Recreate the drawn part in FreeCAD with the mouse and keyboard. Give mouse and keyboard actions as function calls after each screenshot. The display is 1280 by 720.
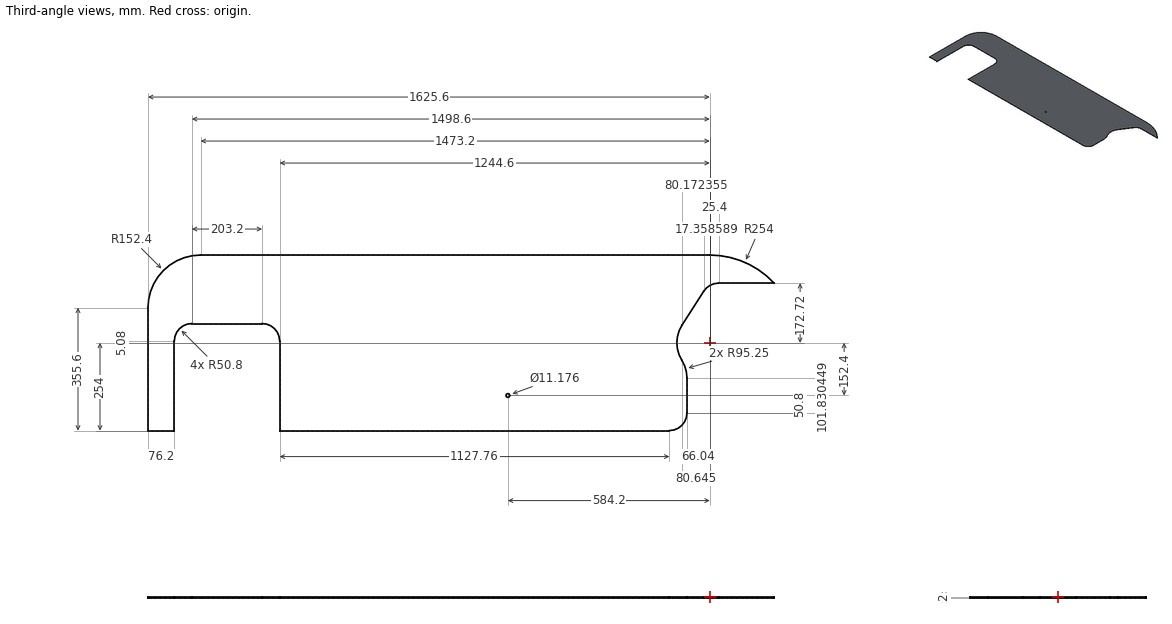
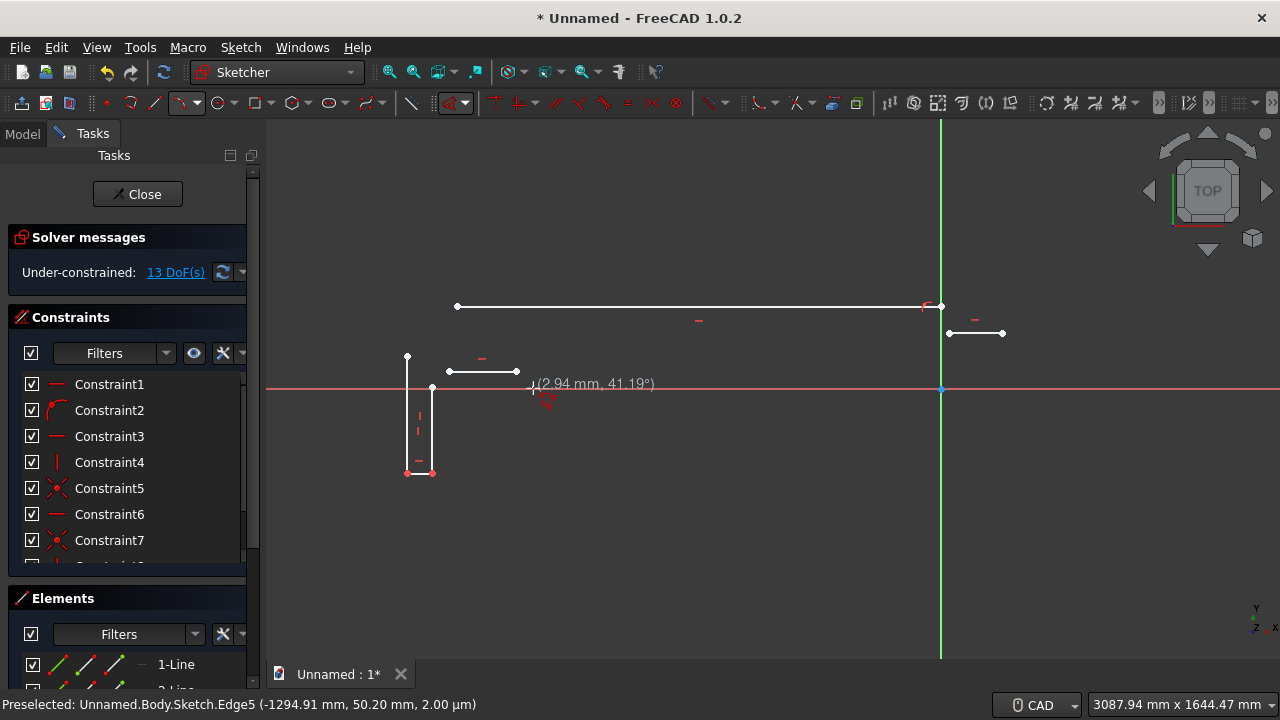
click(533, 473)
click(903, 473)
right_click(903, 473)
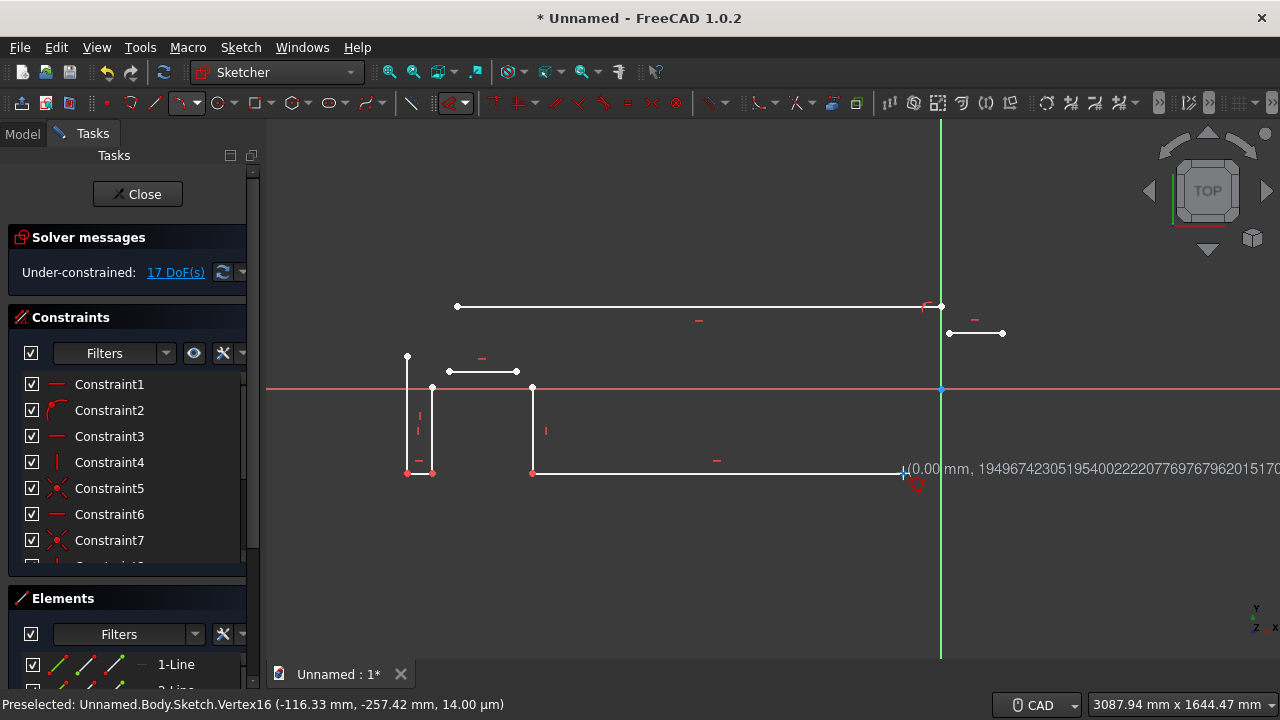
click(156, 104)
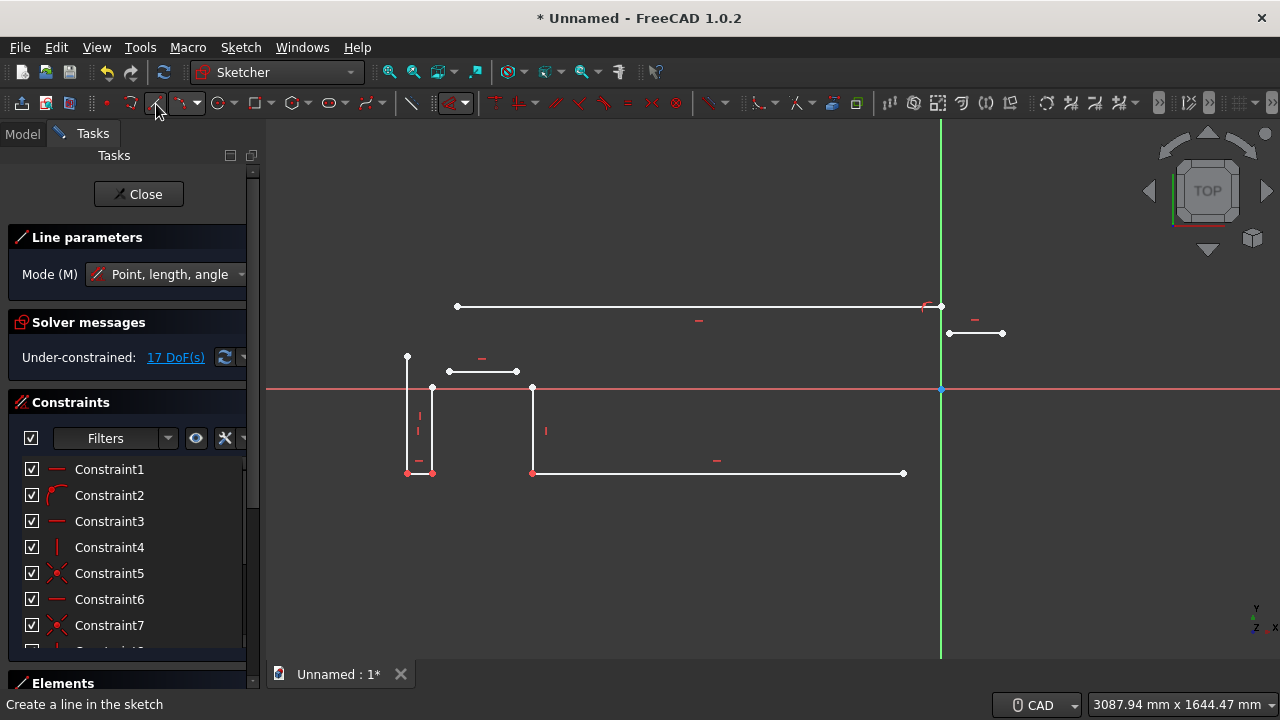
click(920, 456)
click(920, 423)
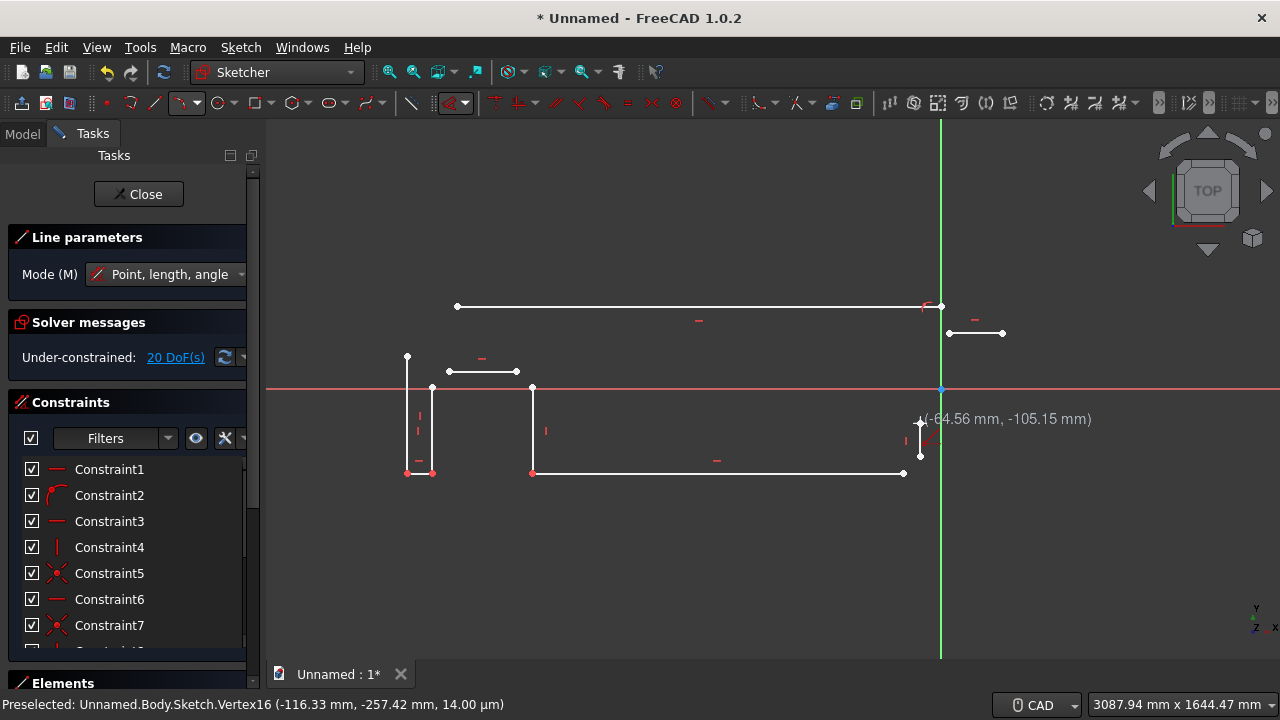
click(915, 373)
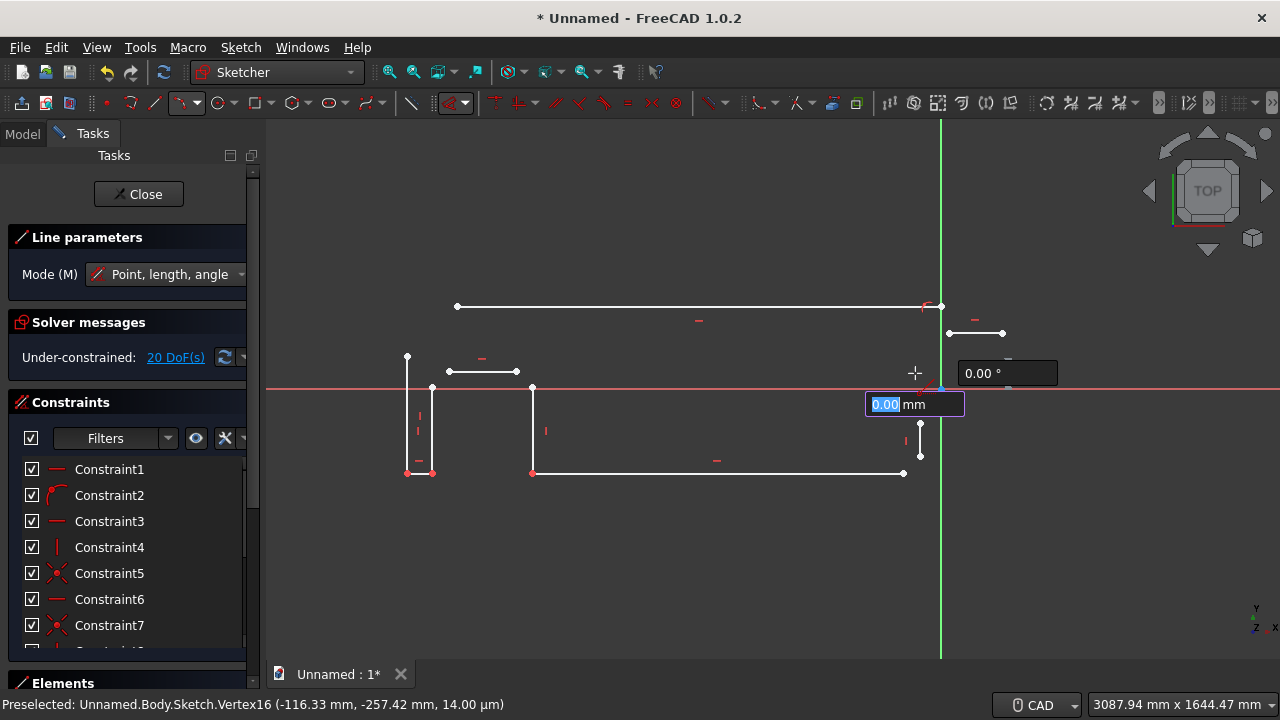
scroll(935, 340, up, 6)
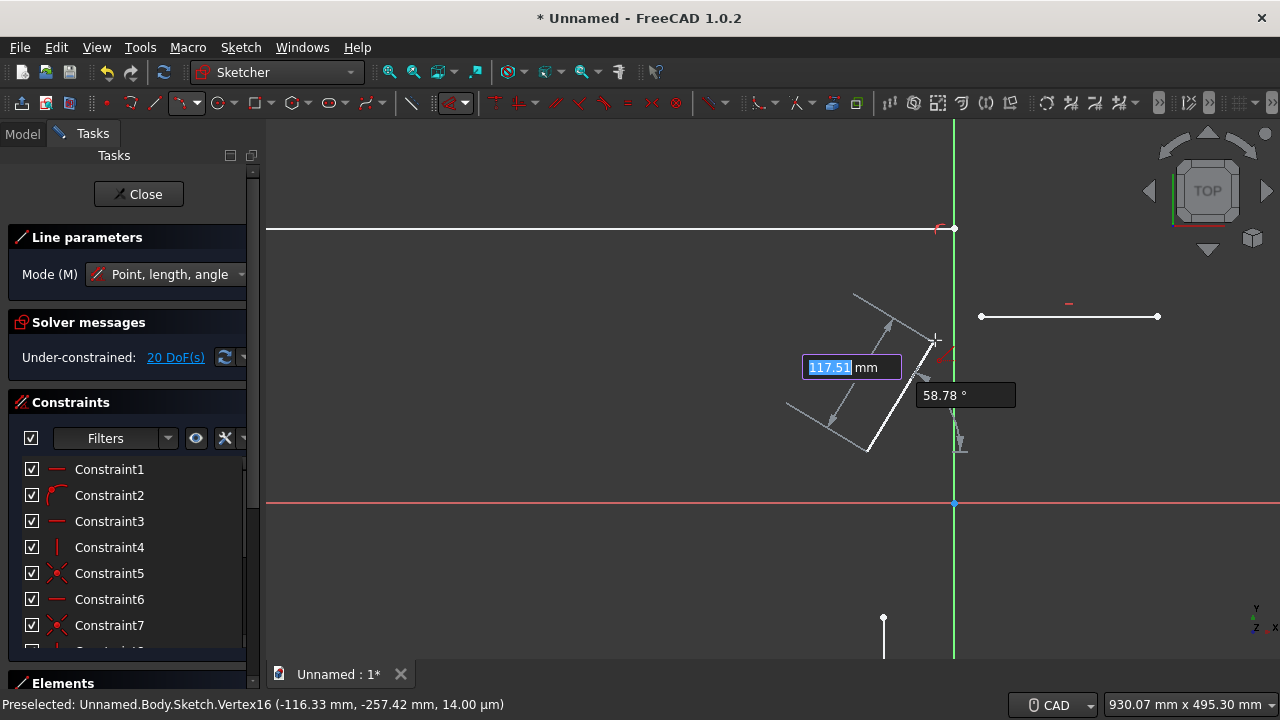
click(935, 340)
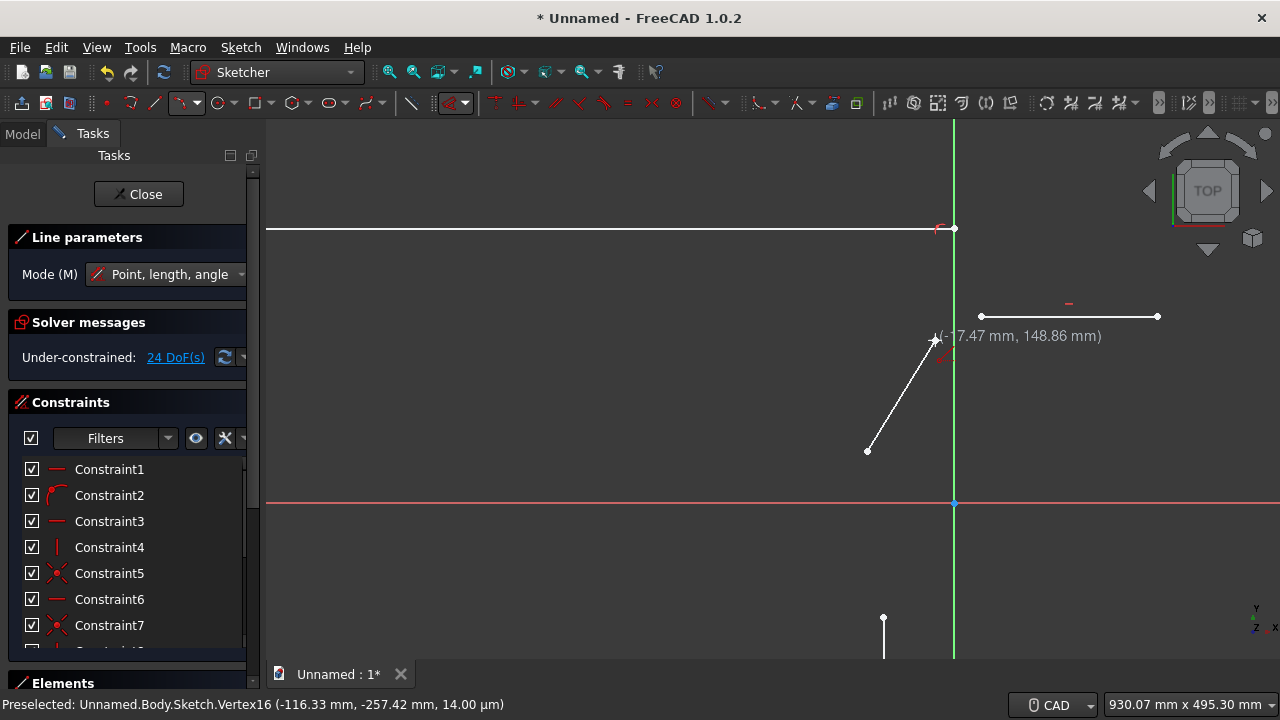
click(180, 104)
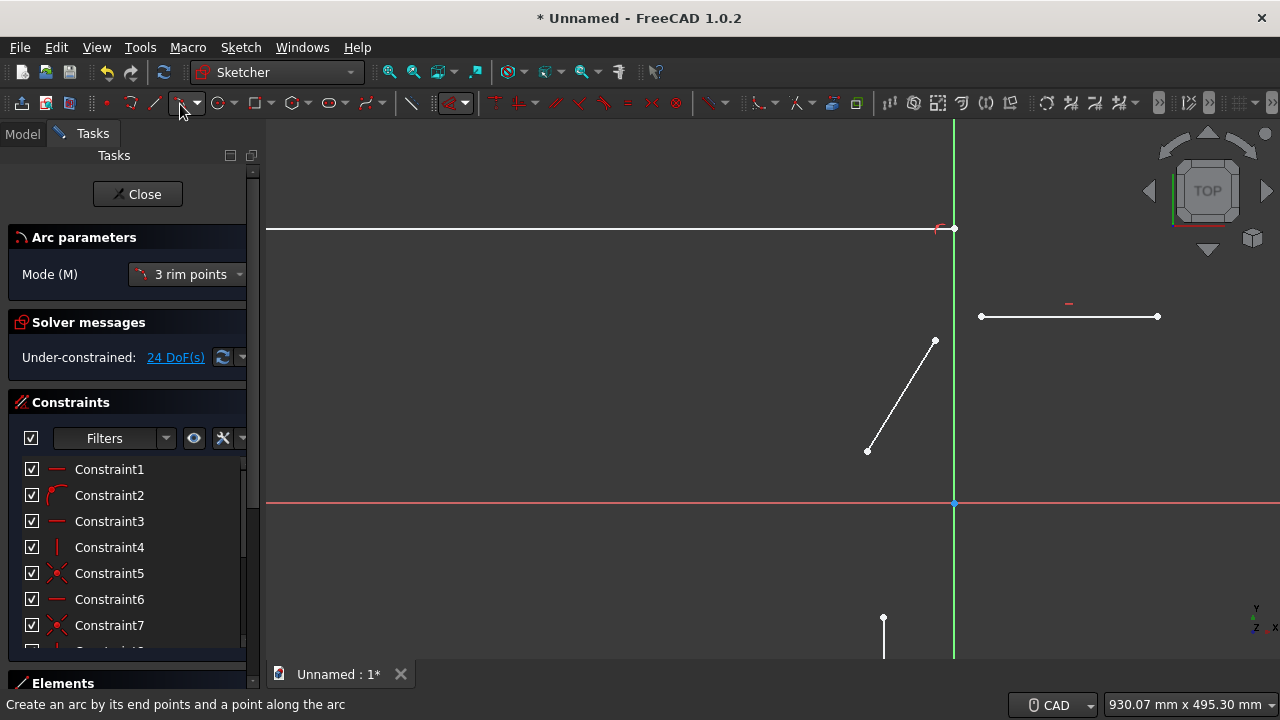
scroll(935, 340, down, 6)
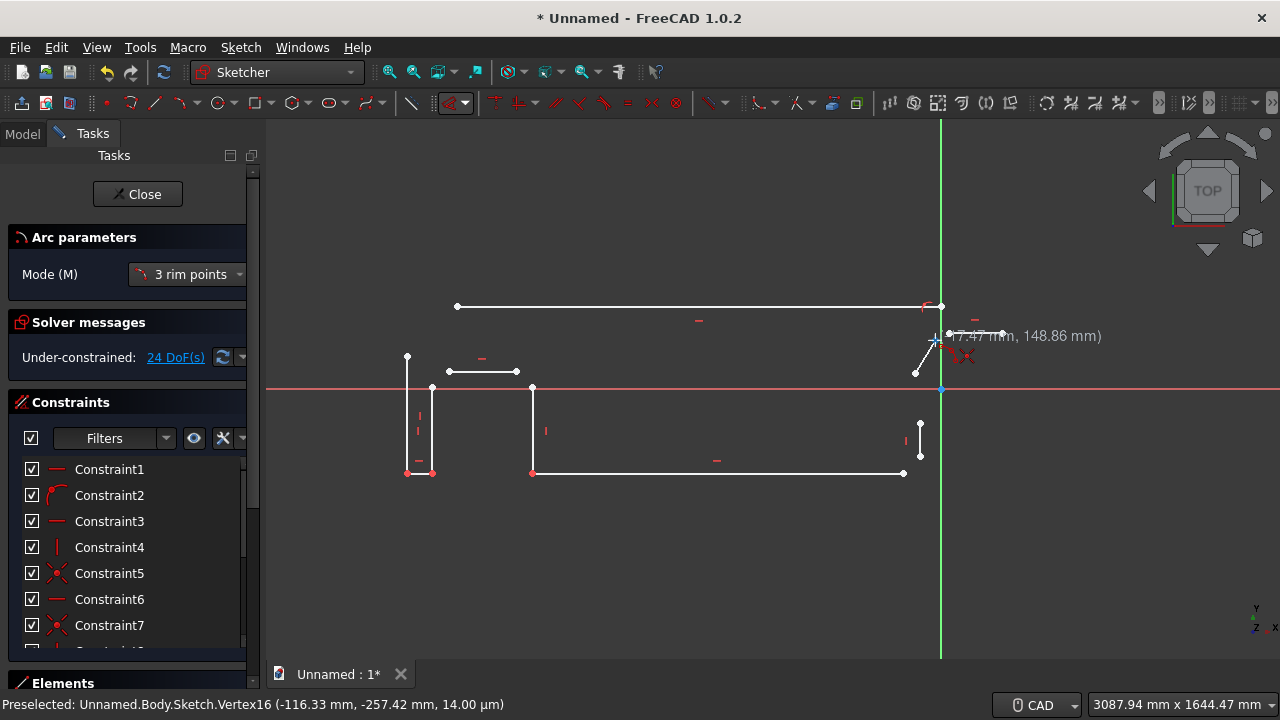
click(1002, 333)
click(941, 307)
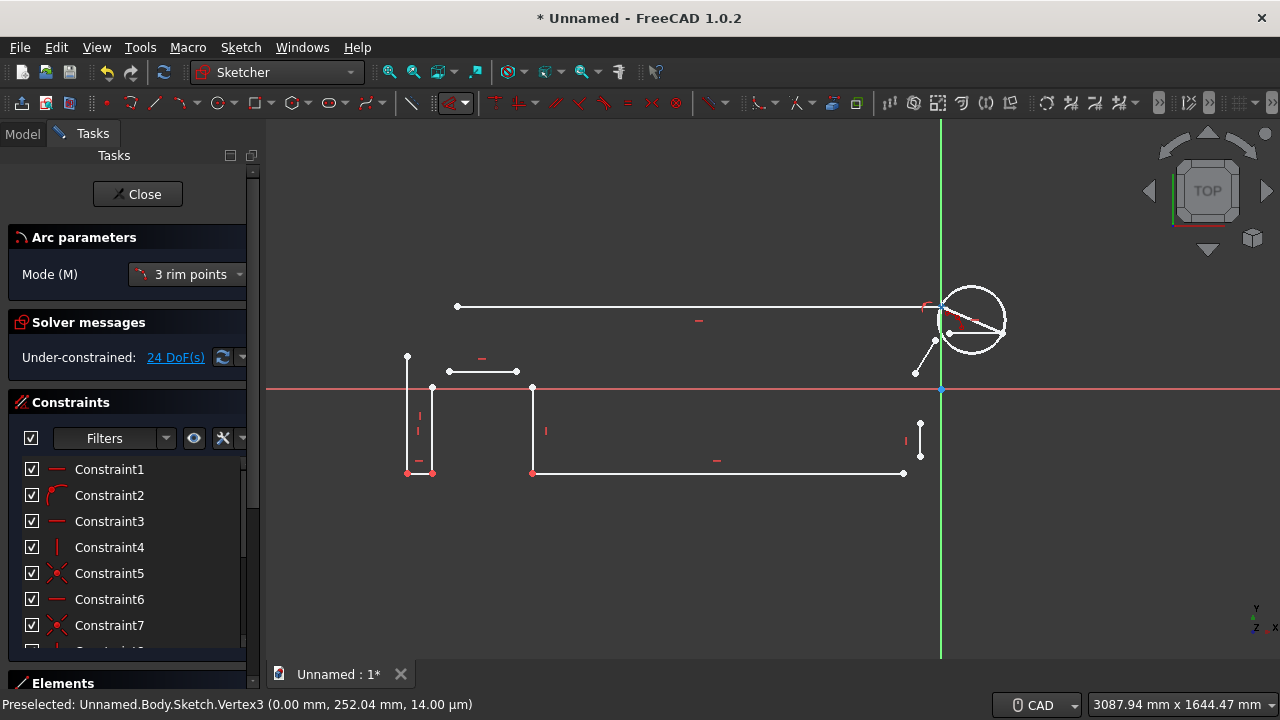
scroll(975, 313, up, 5)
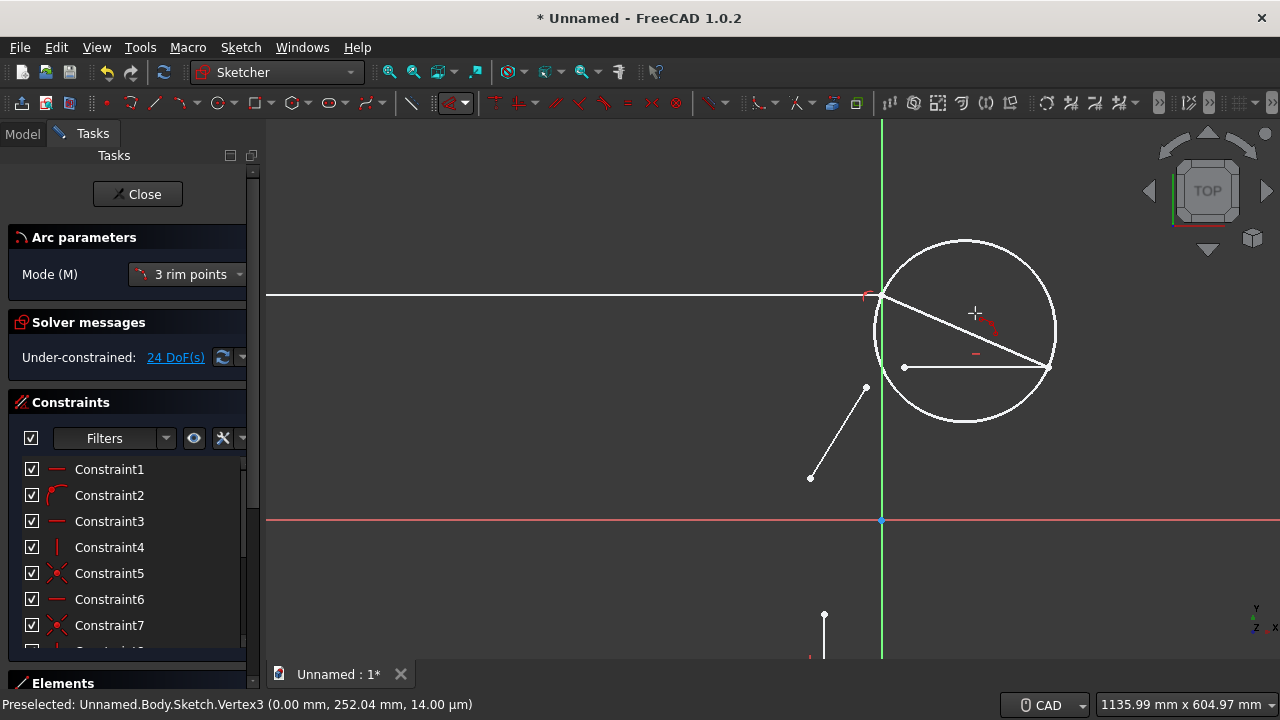
click(973, 312)